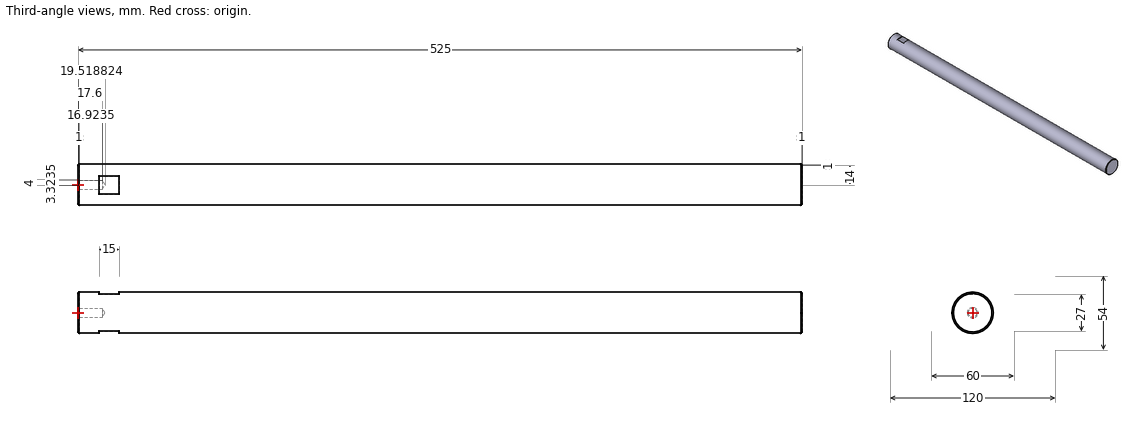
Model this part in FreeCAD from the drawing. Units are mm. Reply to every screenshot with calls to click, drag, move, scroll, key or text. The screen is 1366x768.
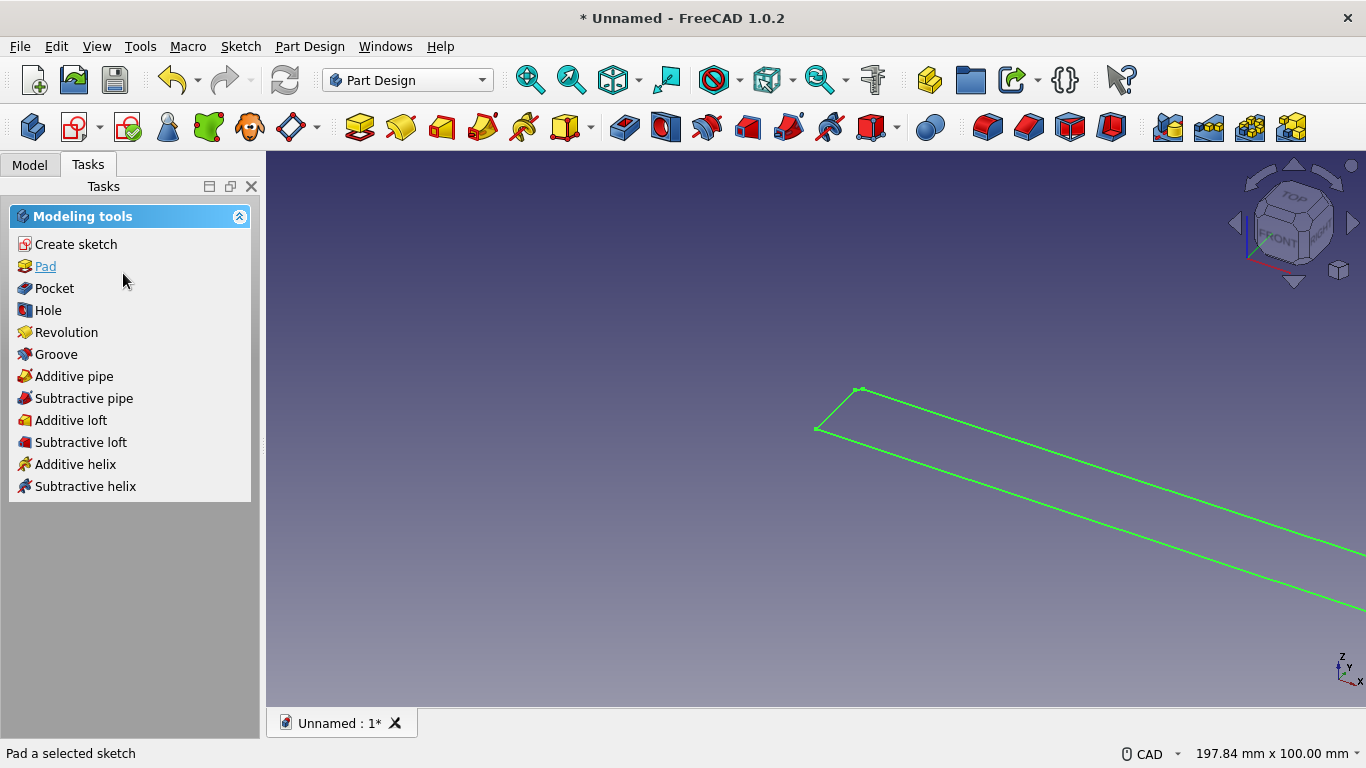
click(401, 128)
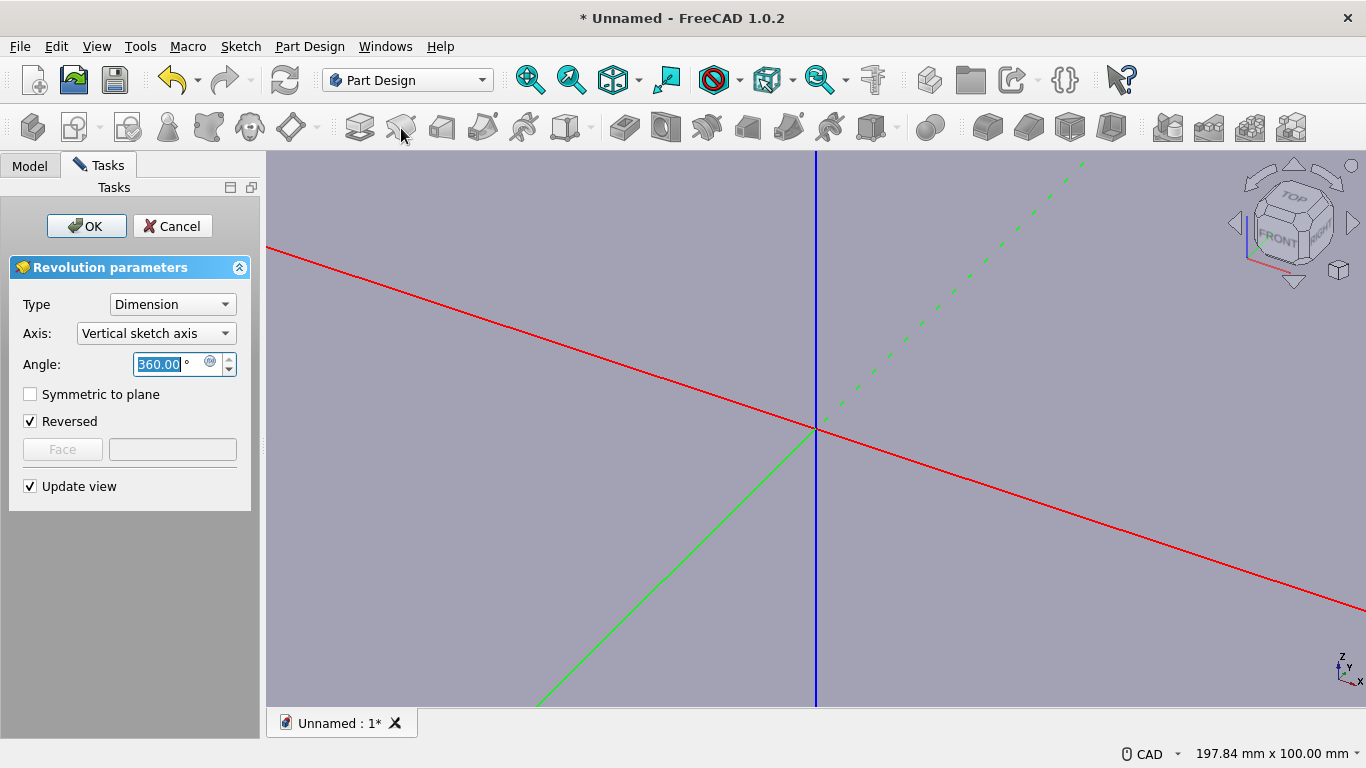
click(157, 334)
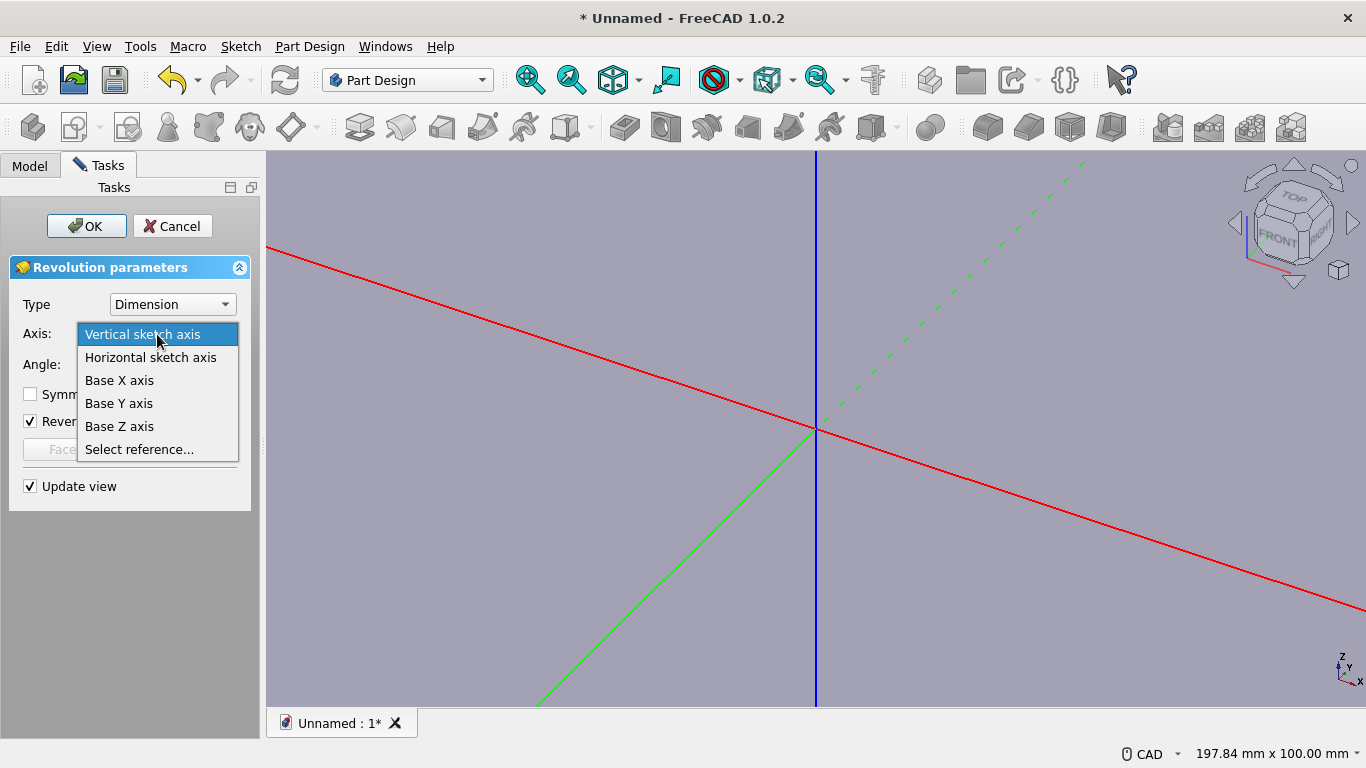
click(156, 358)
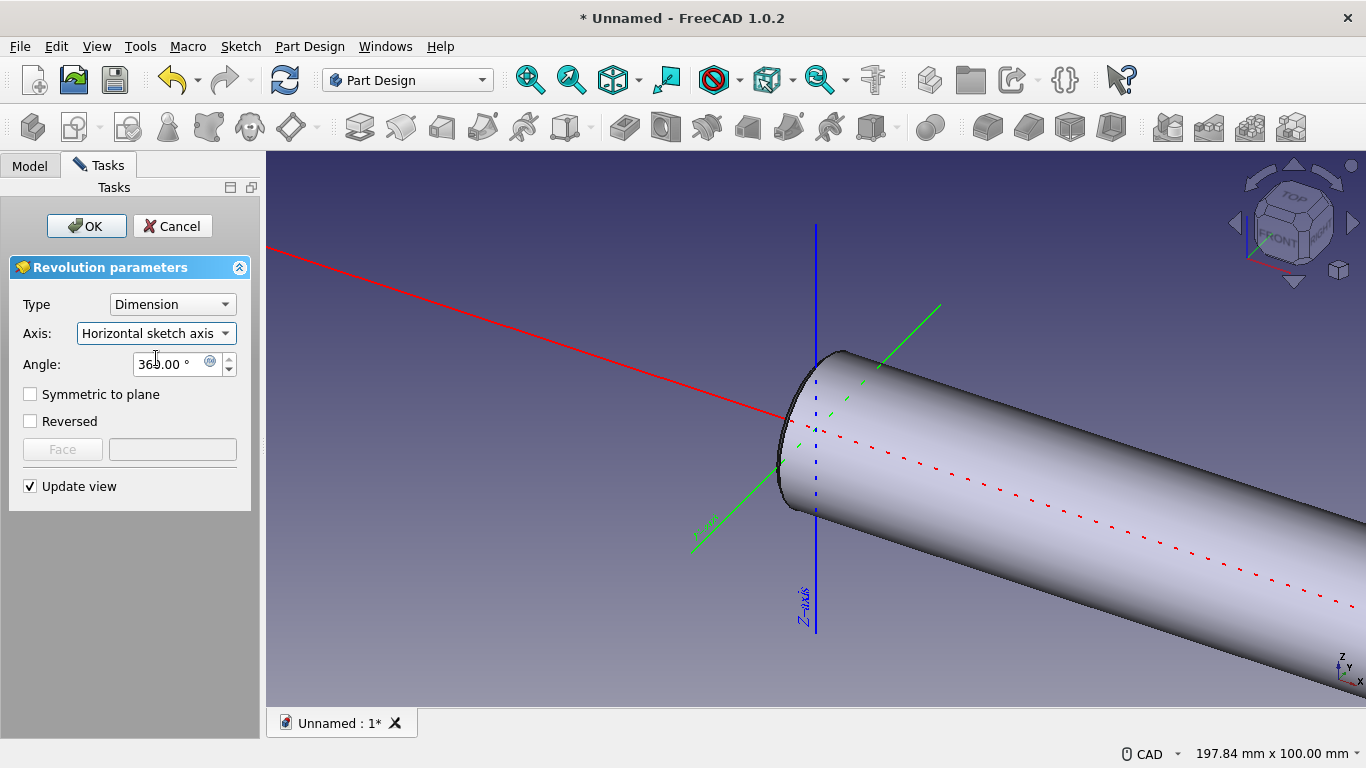
click(87, 226)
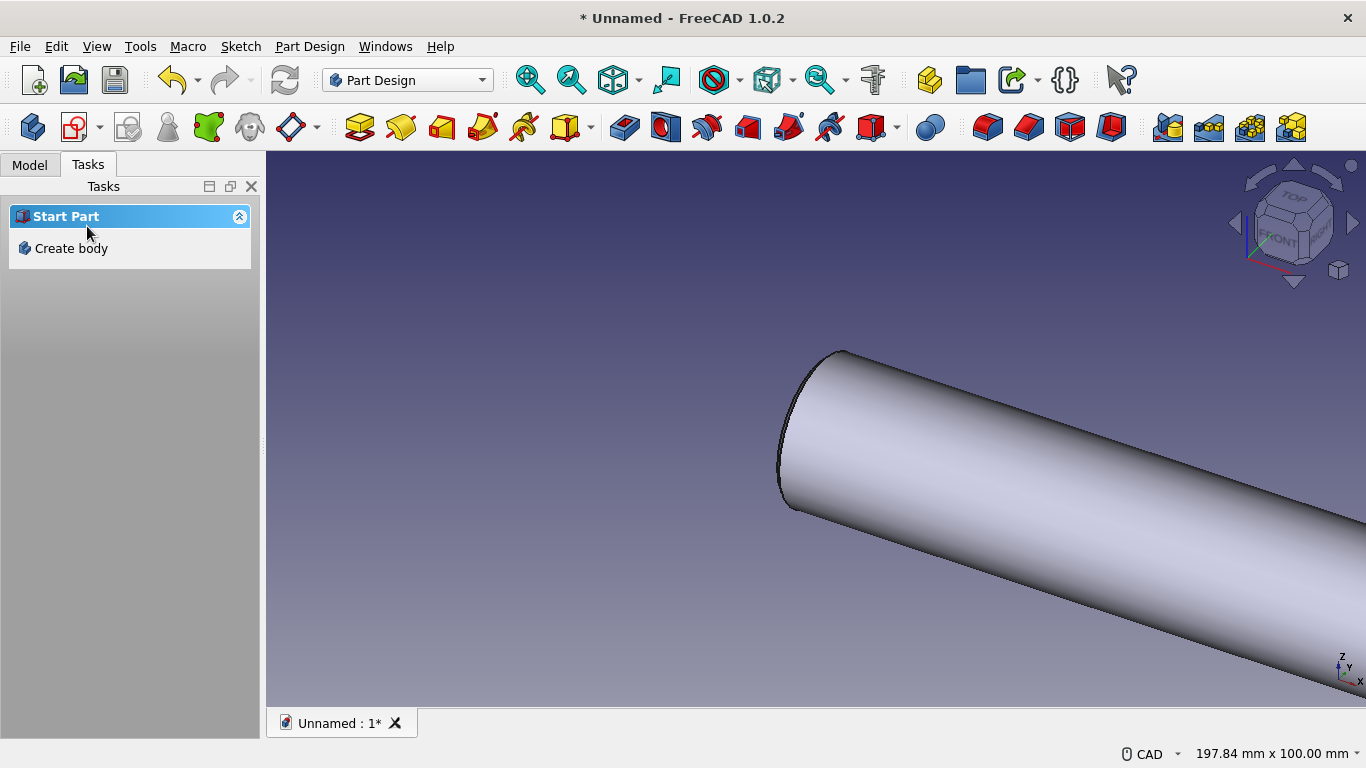
click(531, 80)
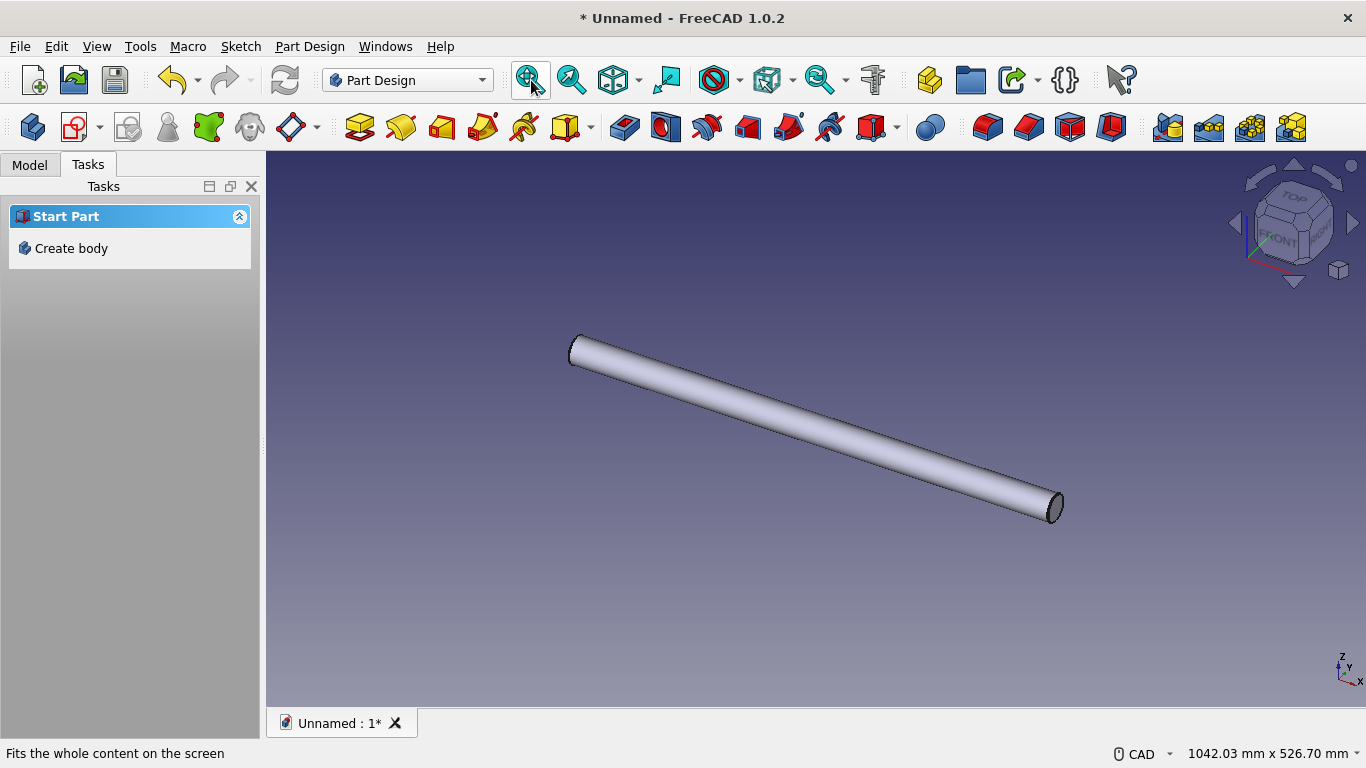
click(74, 128)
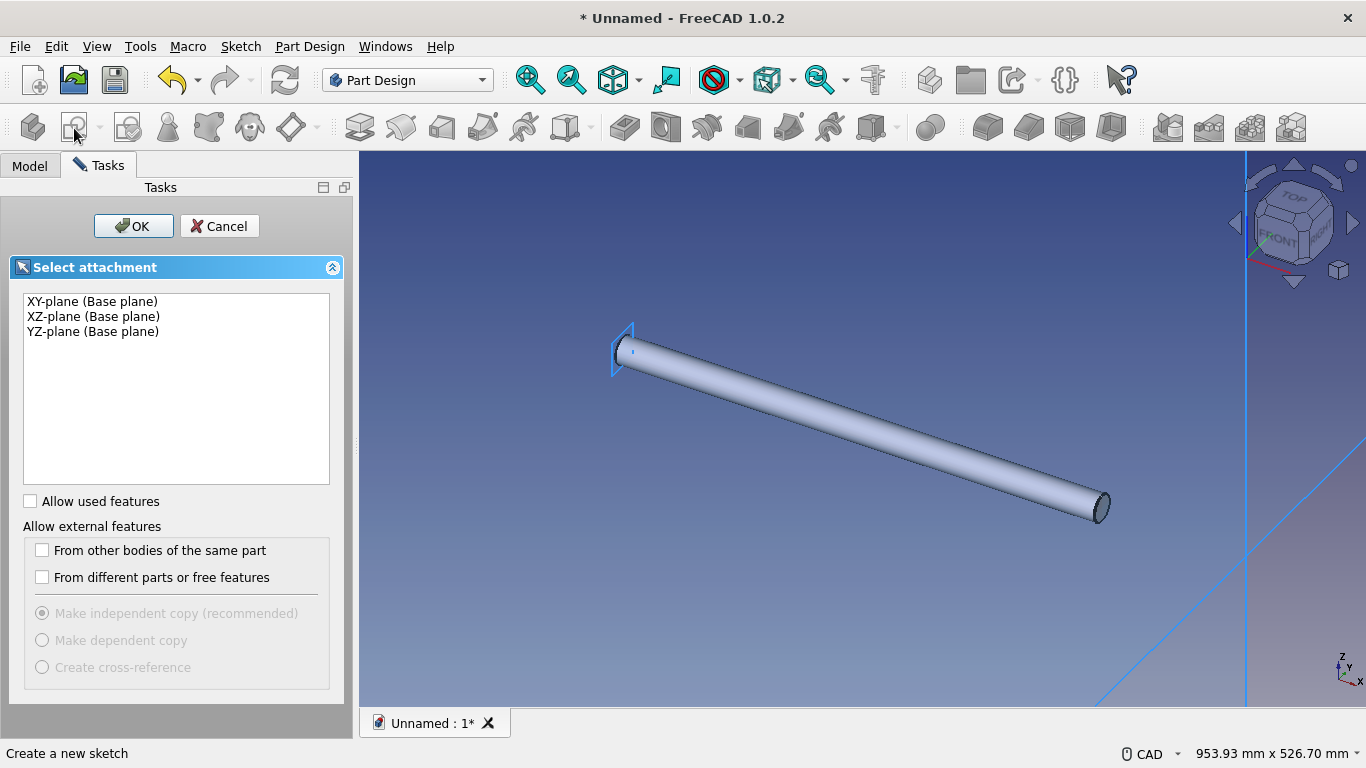
click(84, 302)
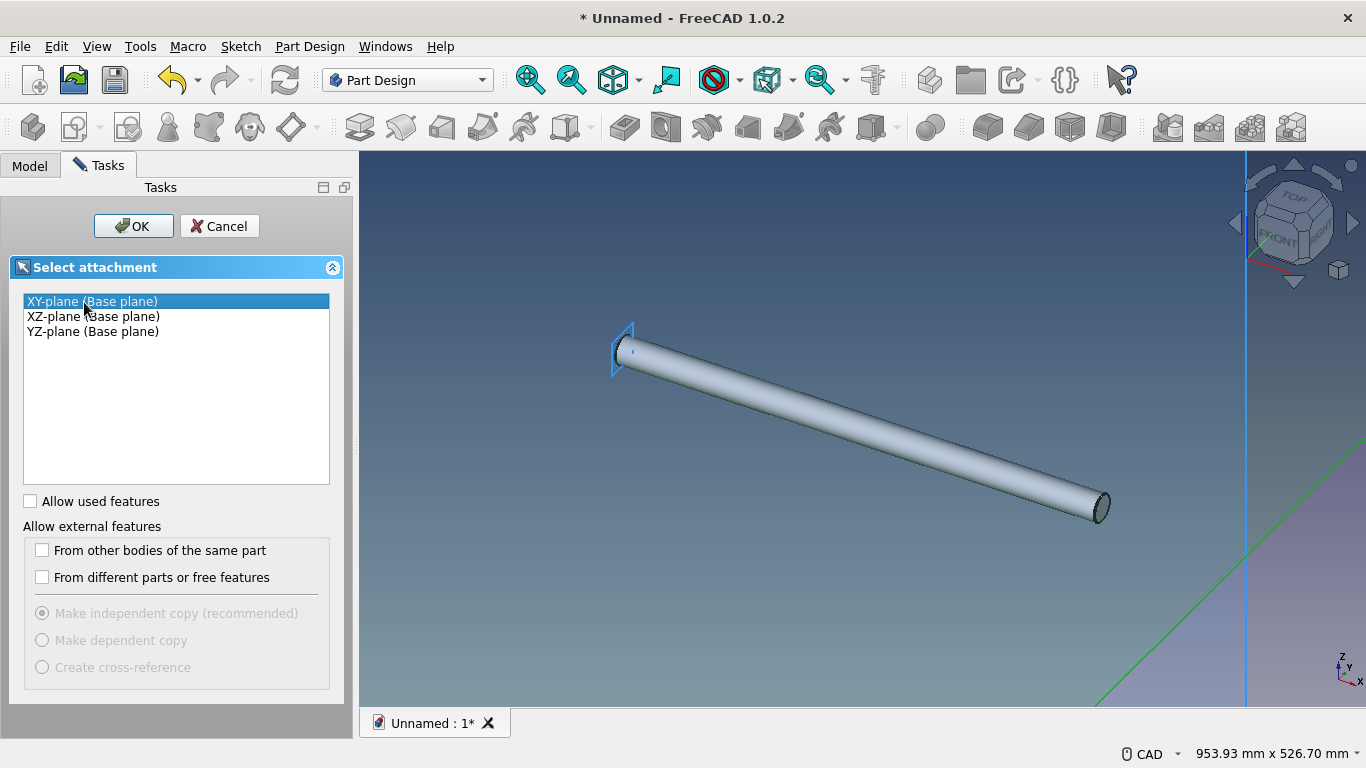
click(134, 226)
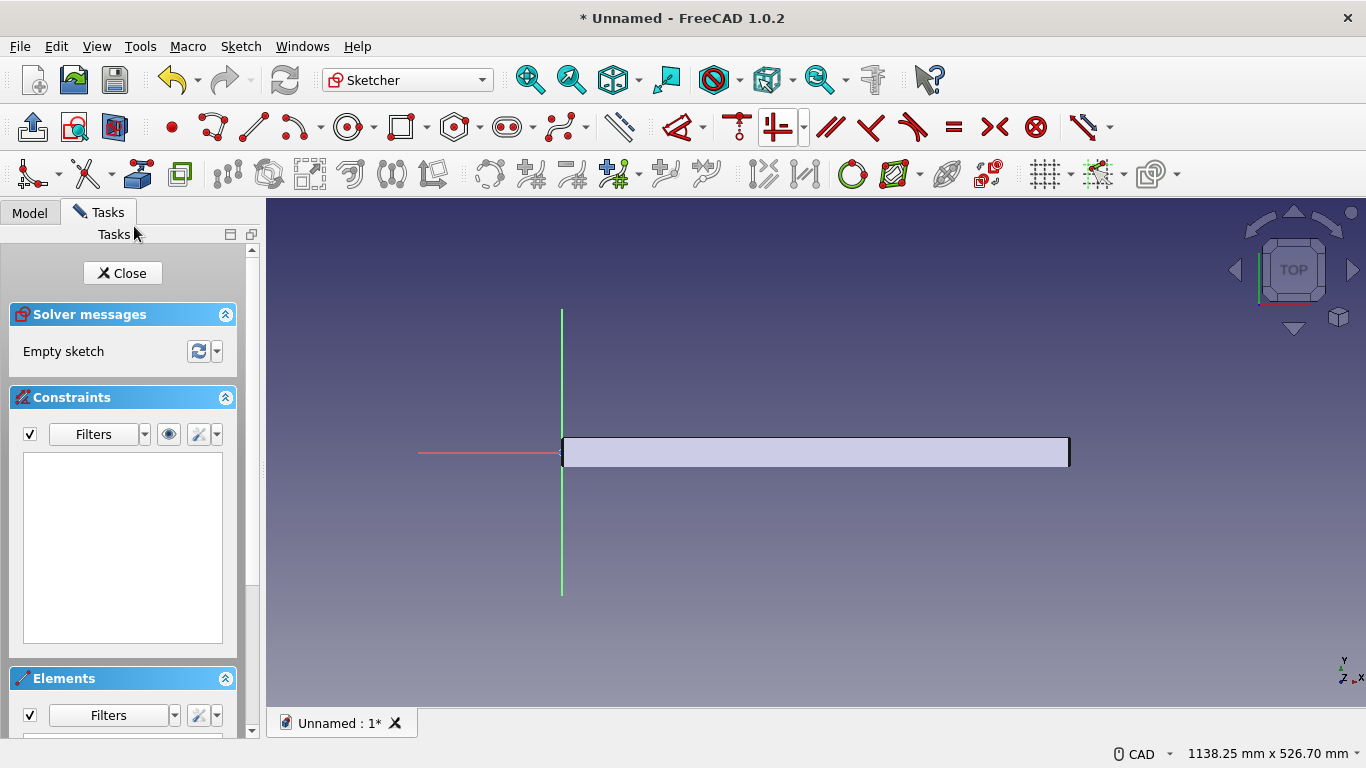
click(115, 128)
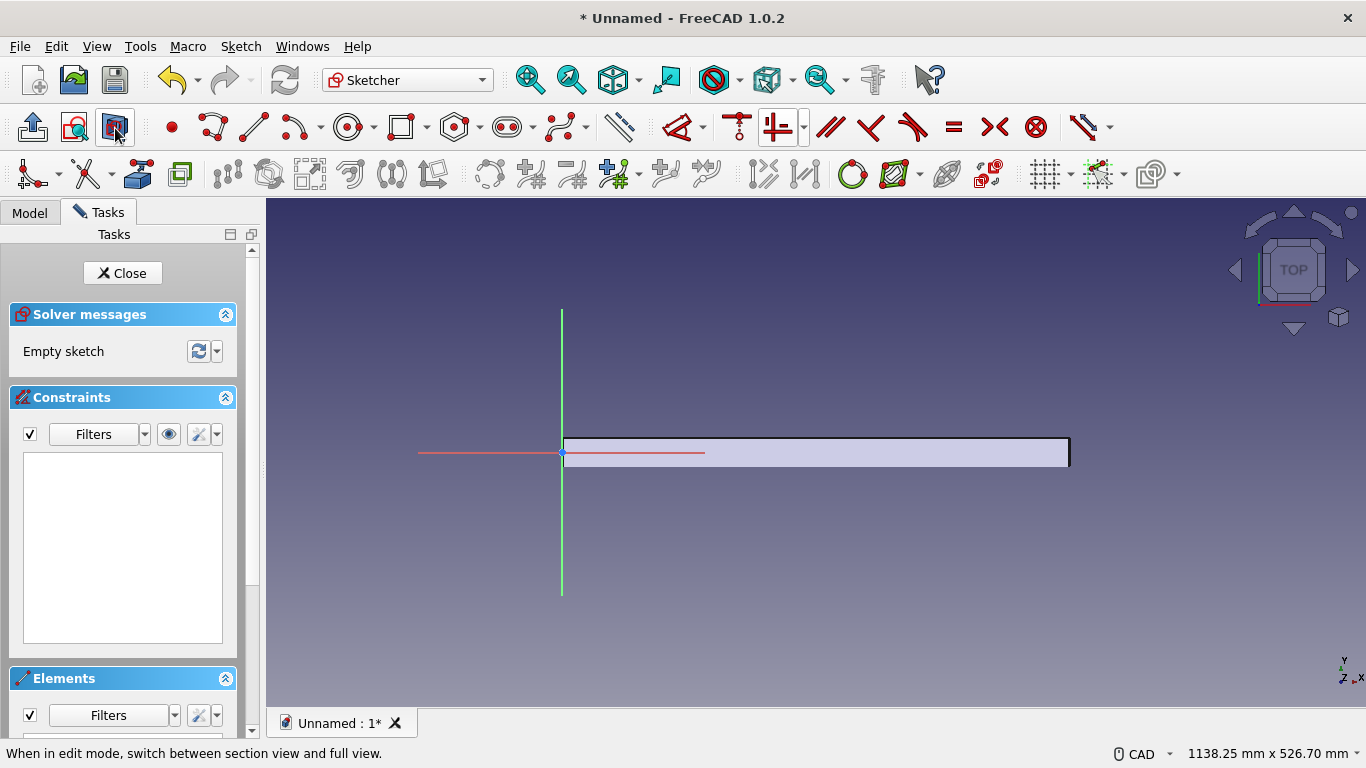
scroll(563, 450, up, 15)